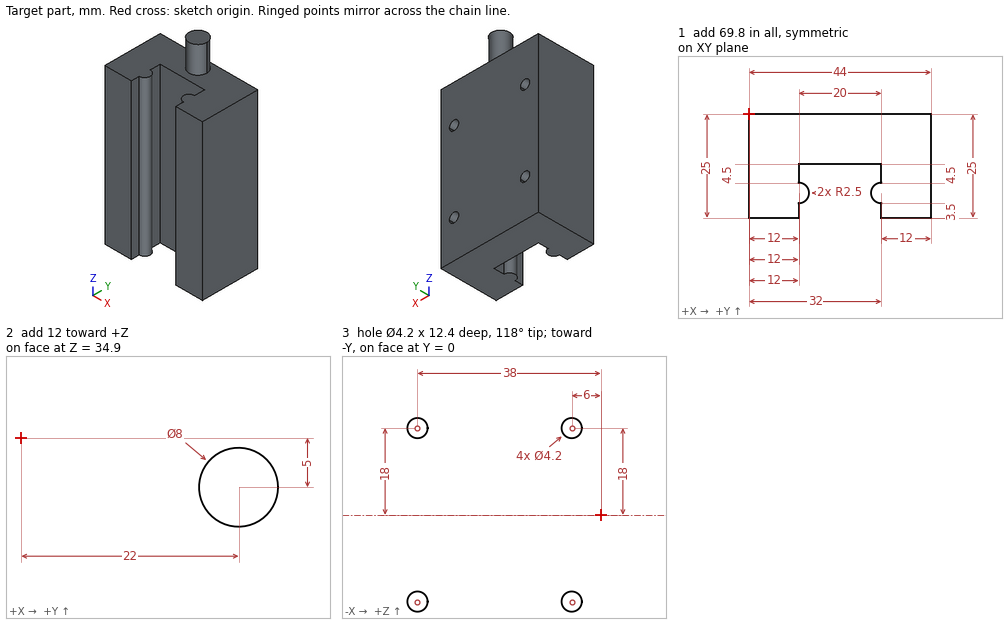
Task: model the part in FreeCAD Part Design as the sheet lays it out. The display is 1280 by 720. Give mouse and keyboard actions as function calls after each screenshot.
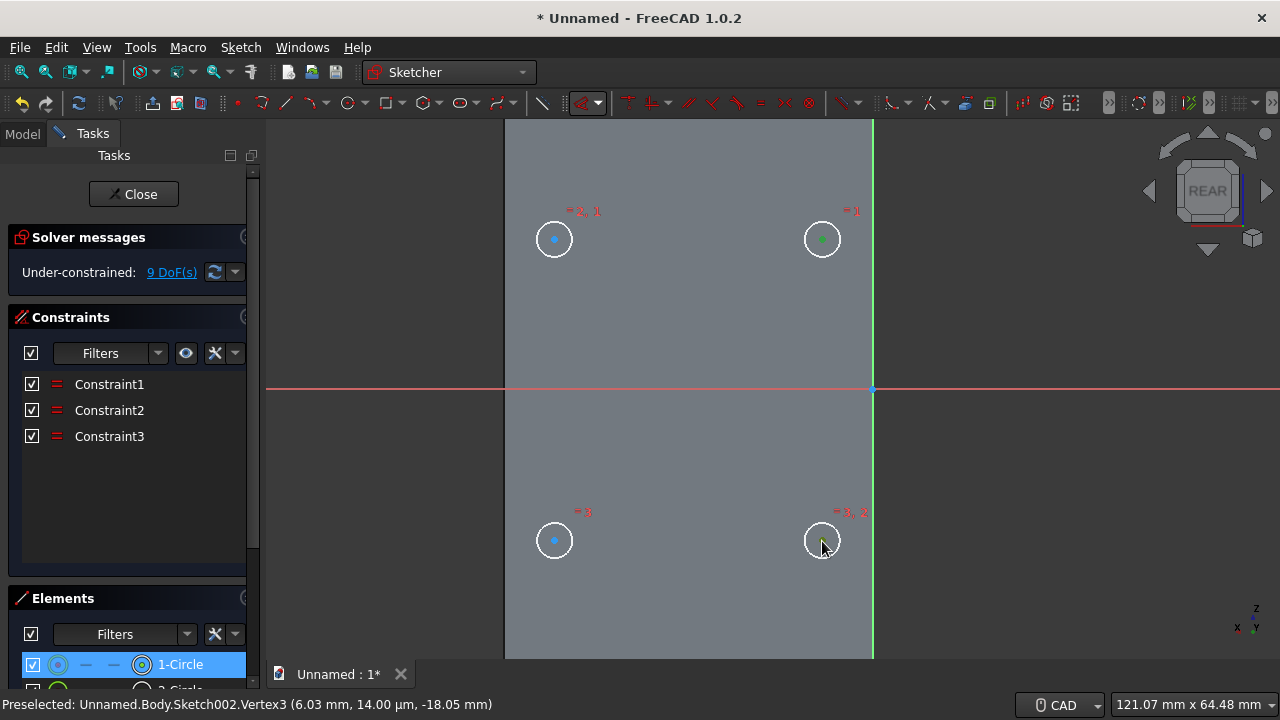
click(353, 389)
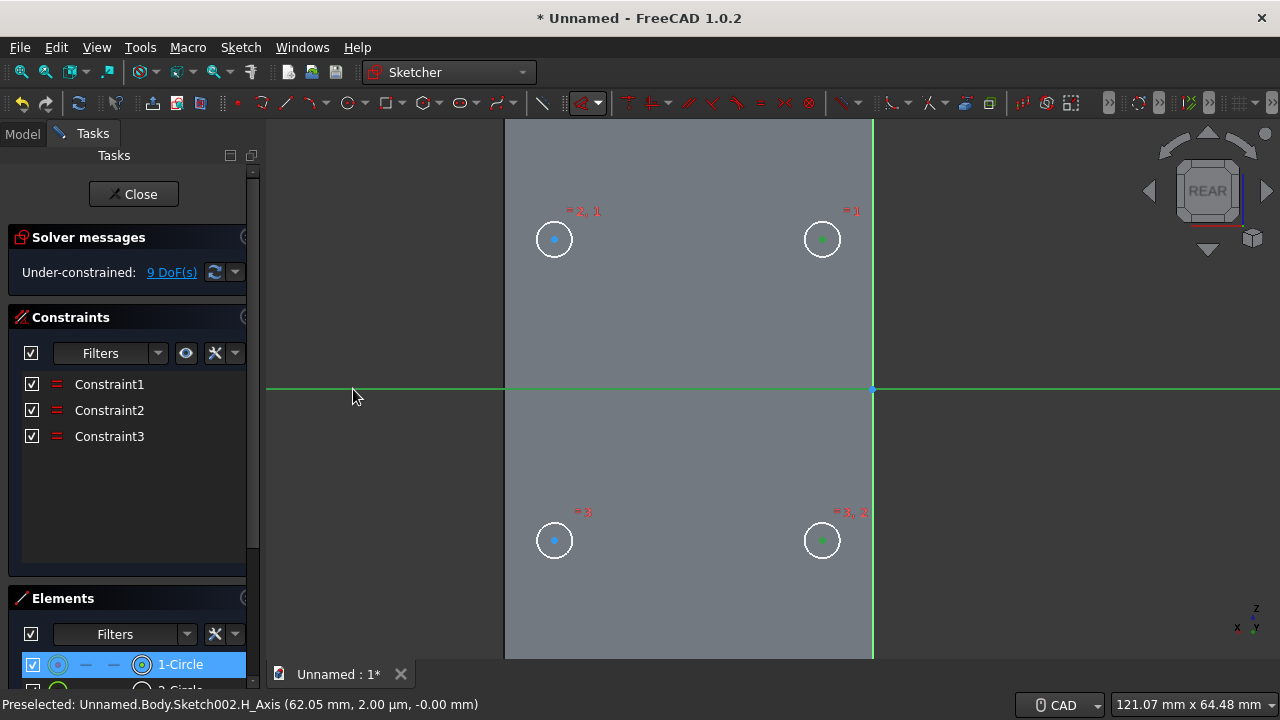
key(s)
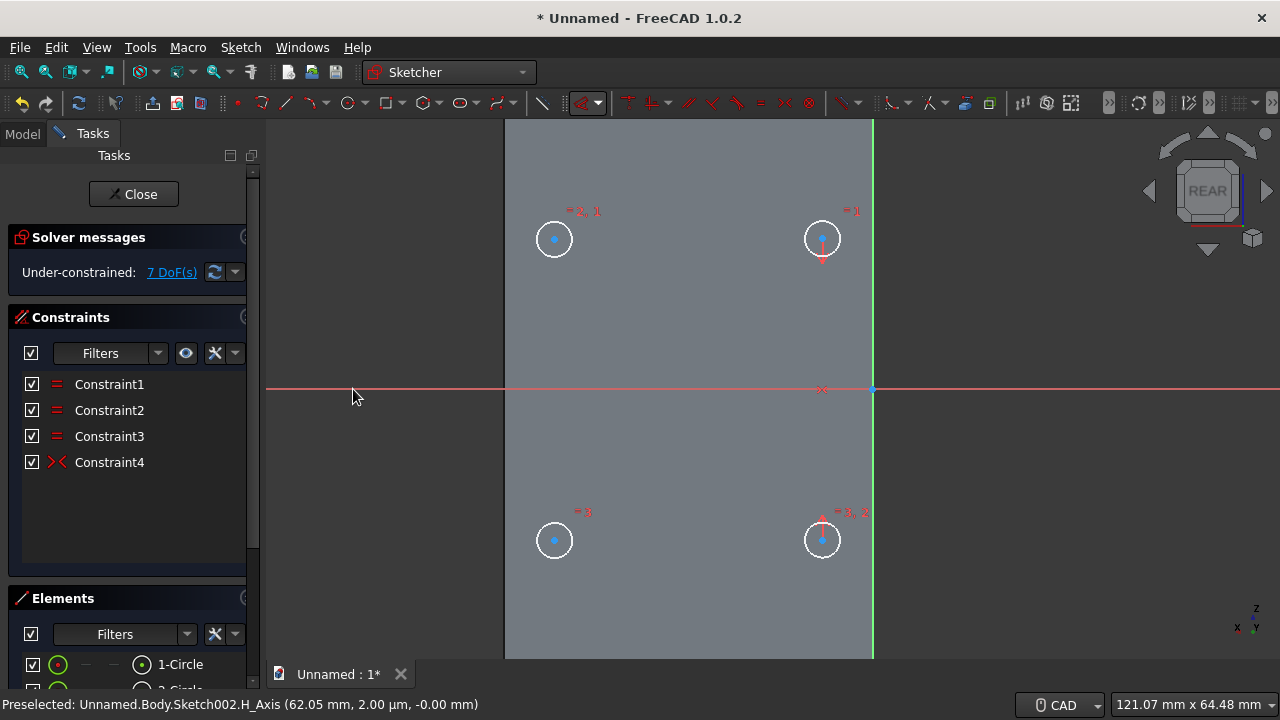
click(554, 239)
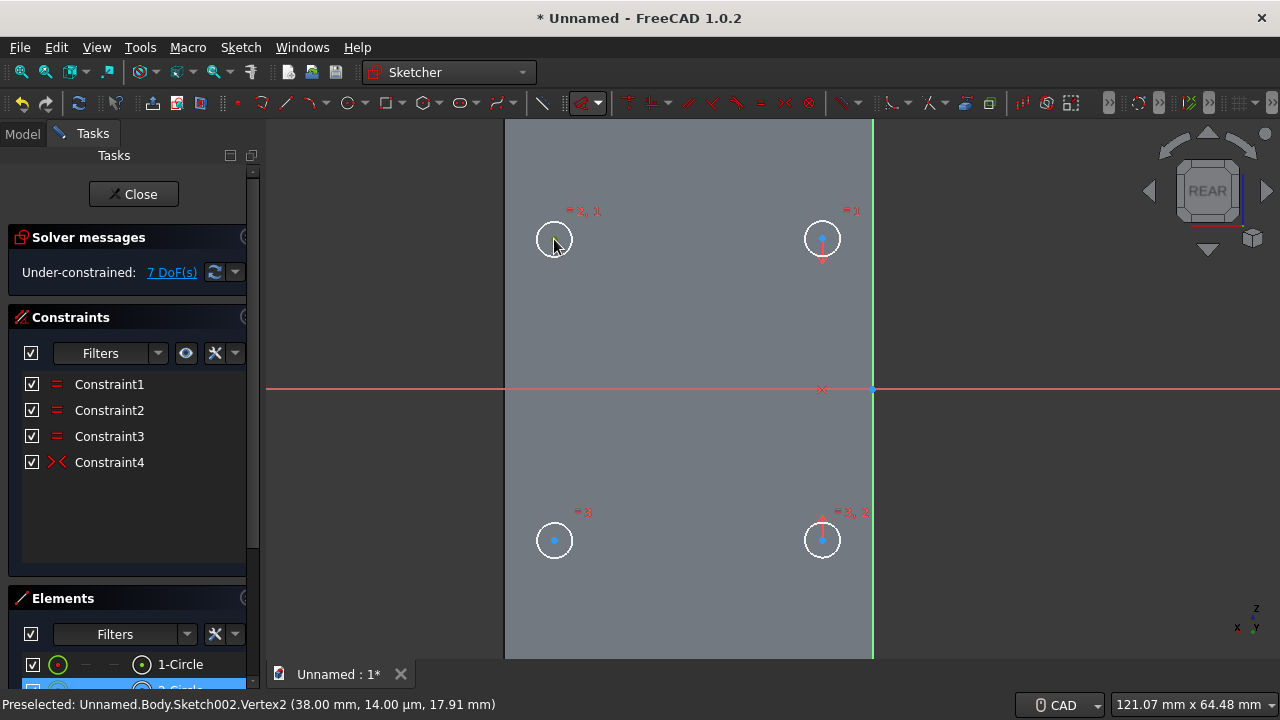
click(555, 541)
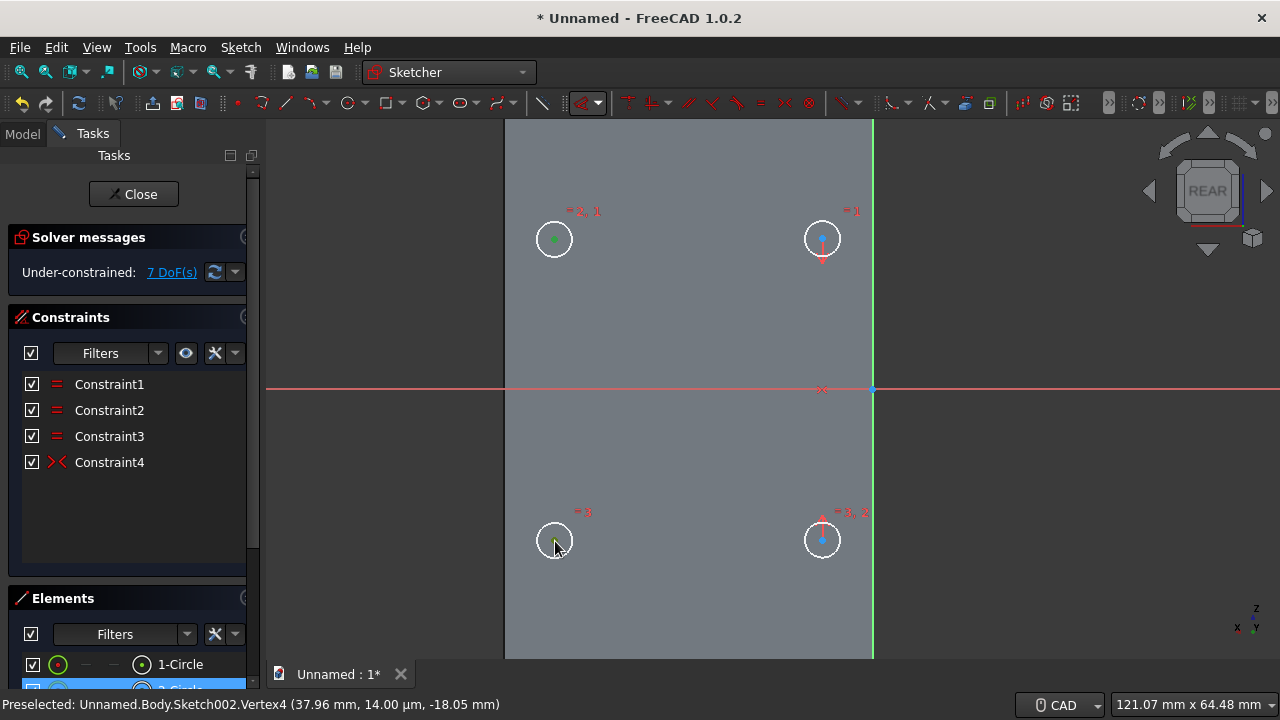
click(353, 389)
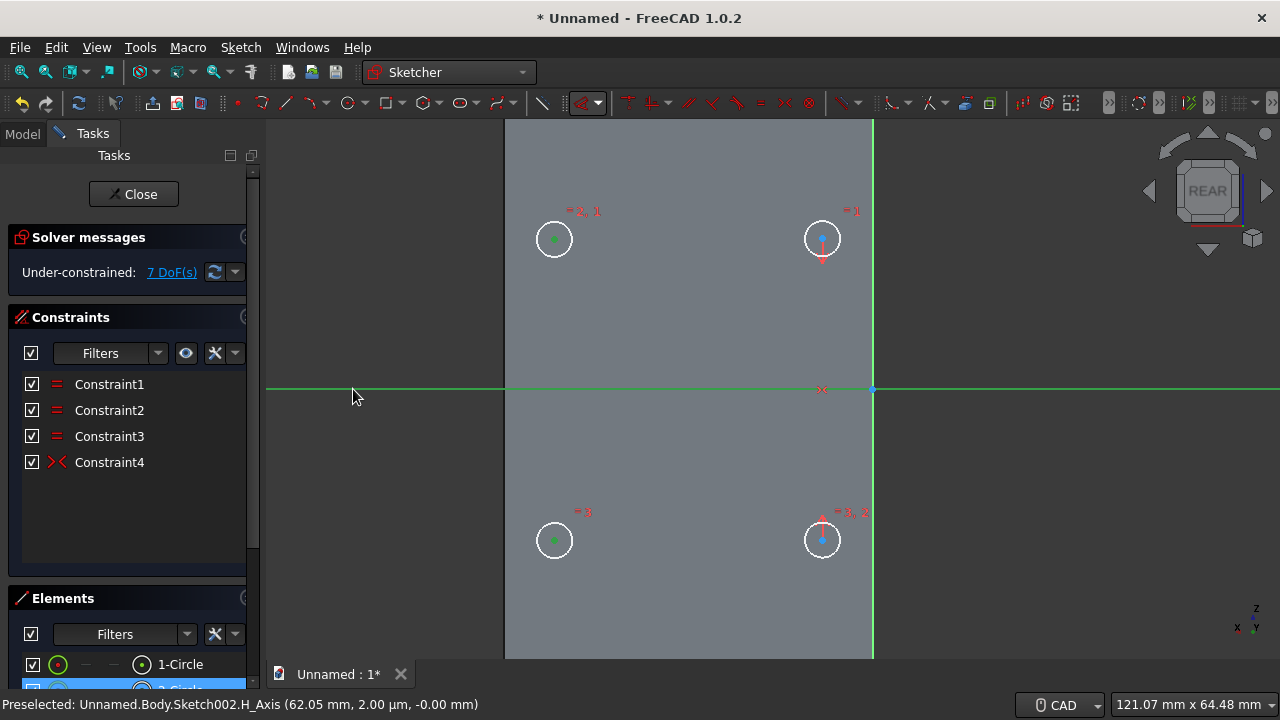
click(786, 104)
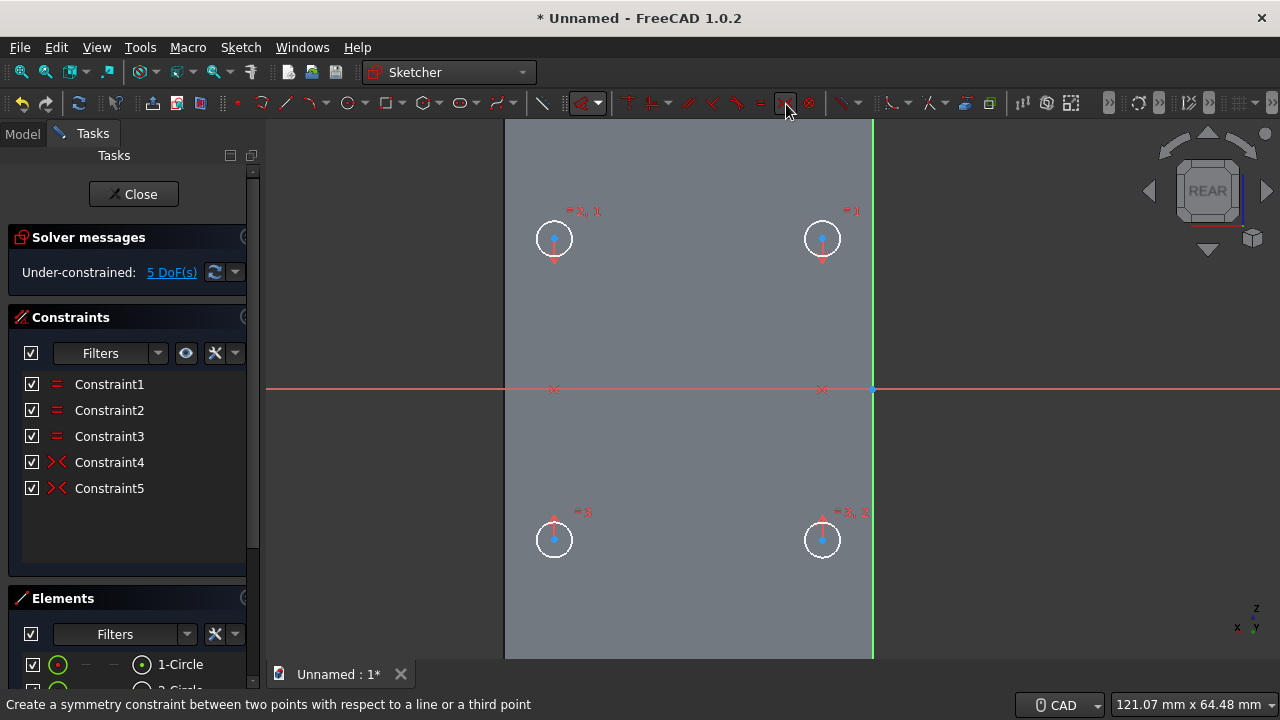
click(835, 226)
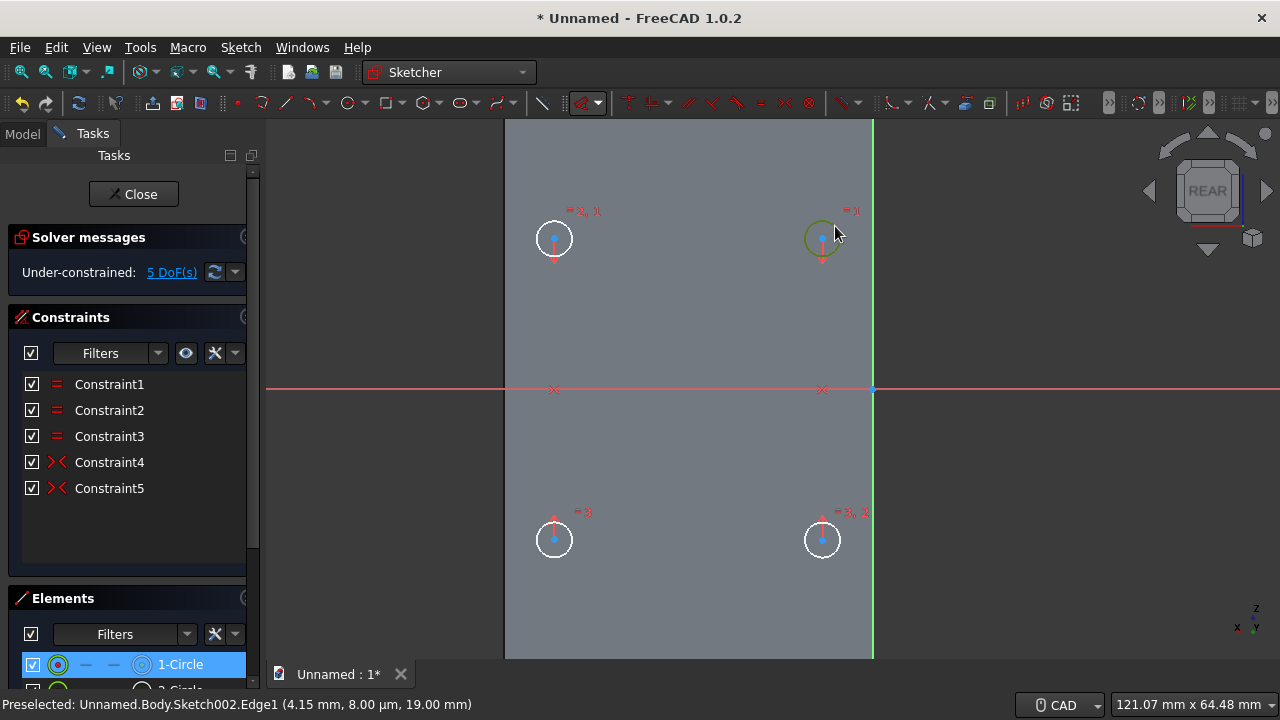
key(k)
key(o)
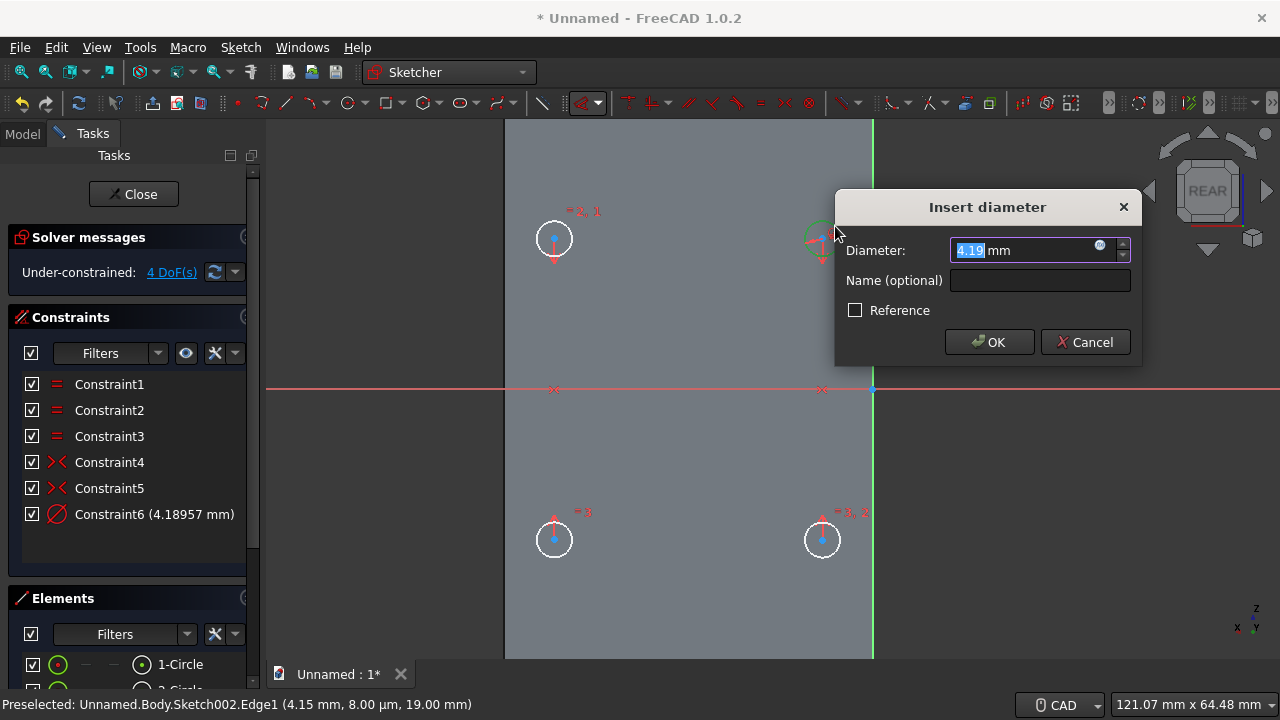
text(4.2)
key(Return)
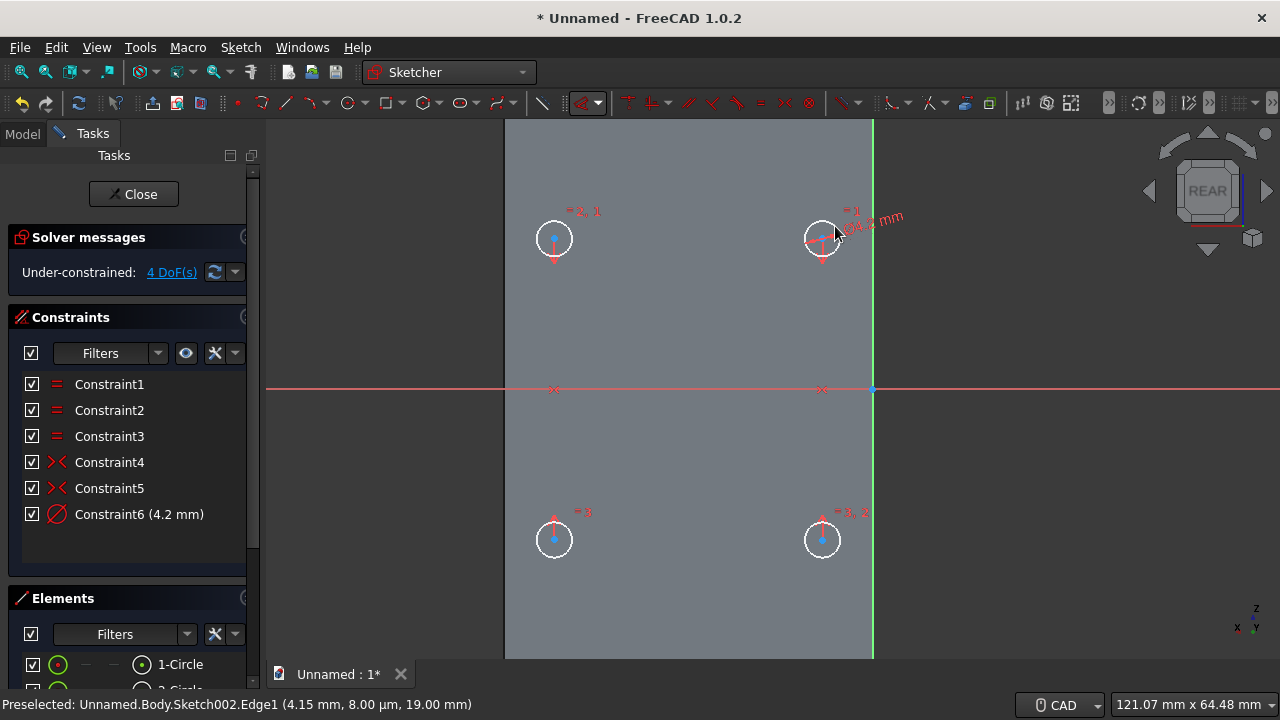
click(823, 239)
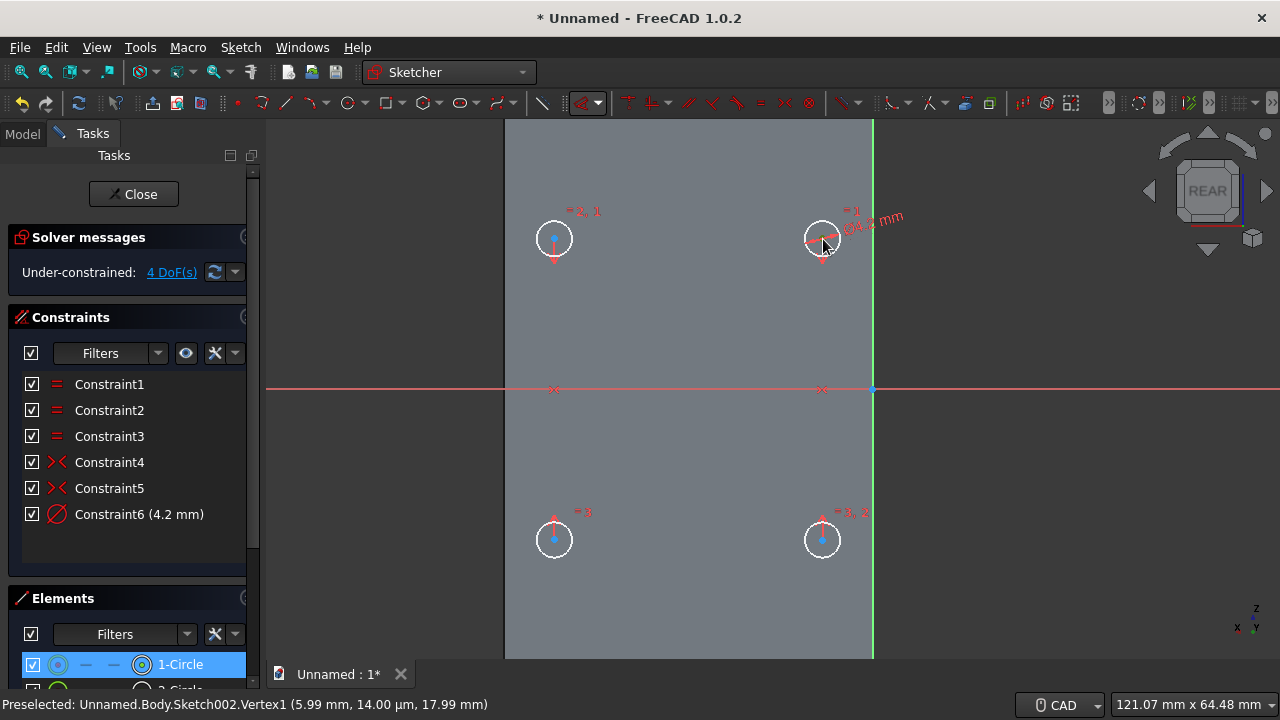
click(600, 104)